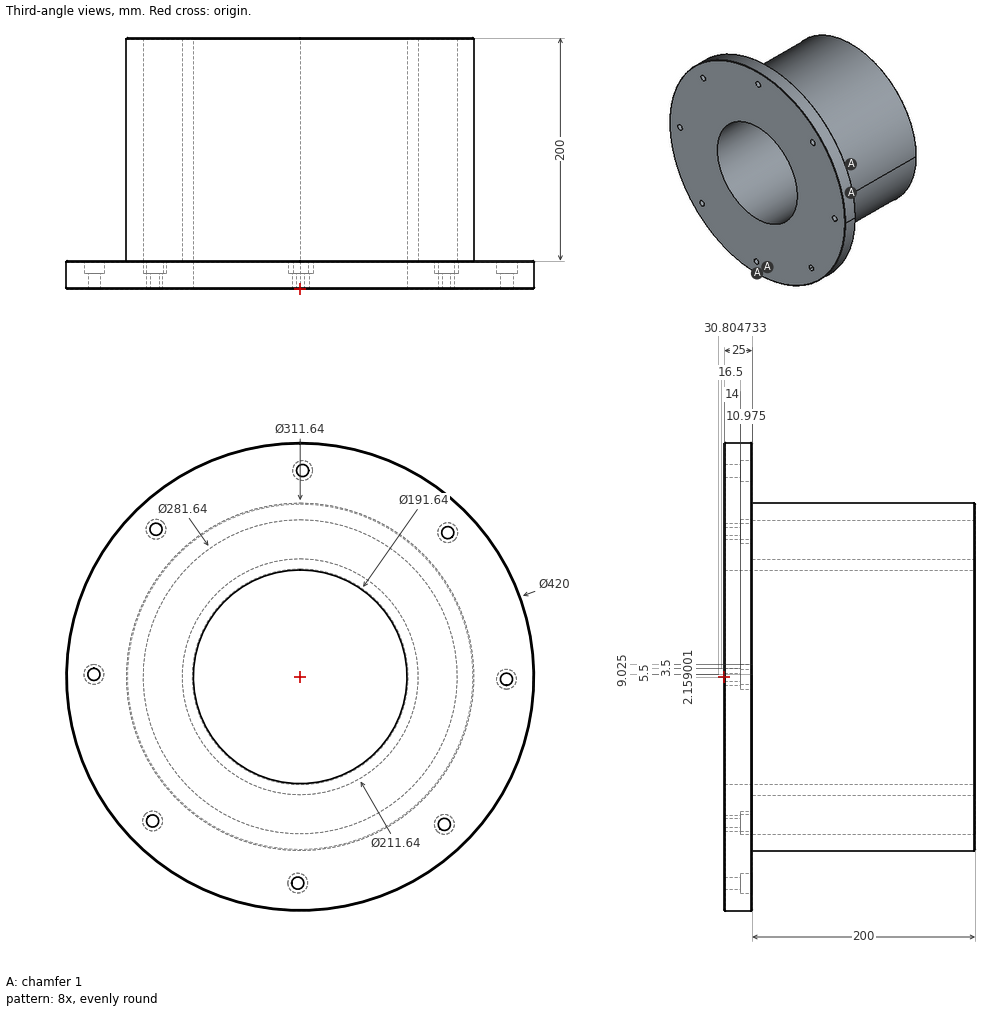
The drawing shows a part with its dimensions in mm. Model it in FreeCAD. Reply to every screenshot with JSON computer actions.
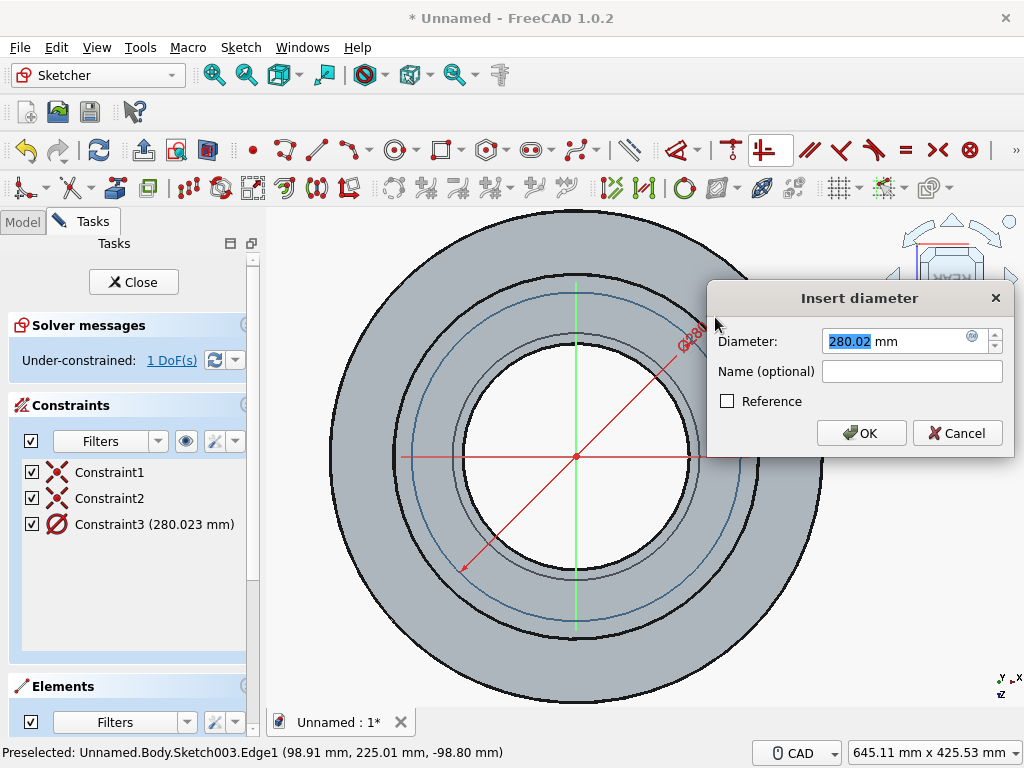
{"action": "type", "text": "281.64"}
{"action": "key", "text": "Return"}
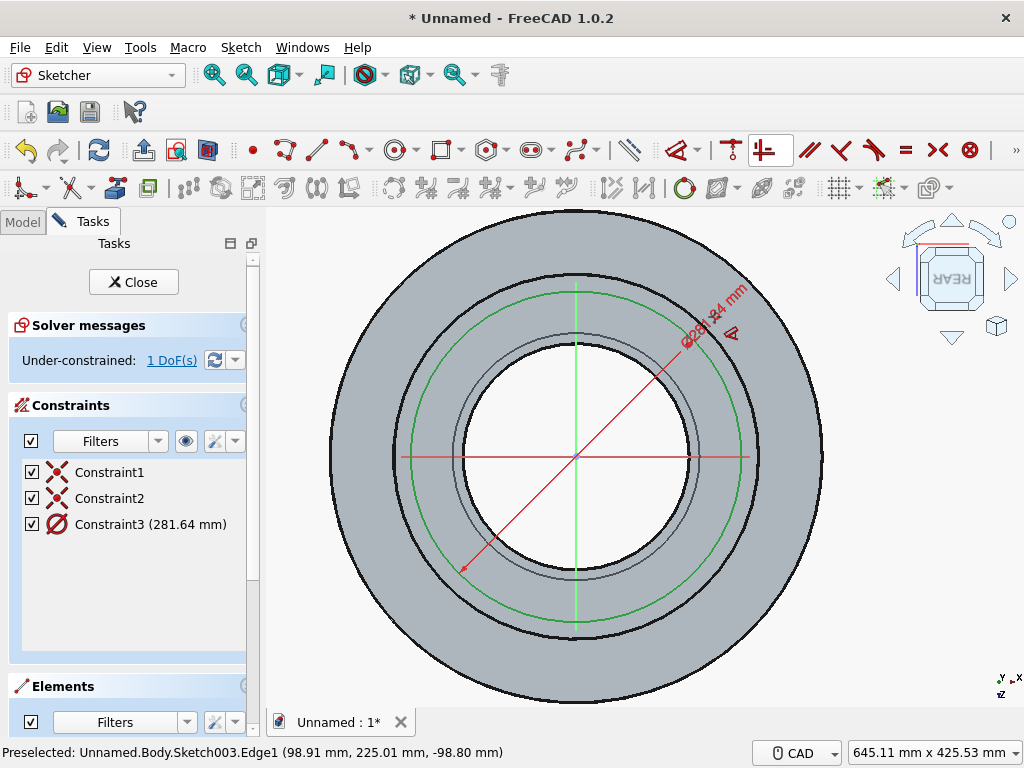
{"action": "left_click", "coordinate": [663, 369]}
{"action": "left_click", "coordinate": [747, 406]}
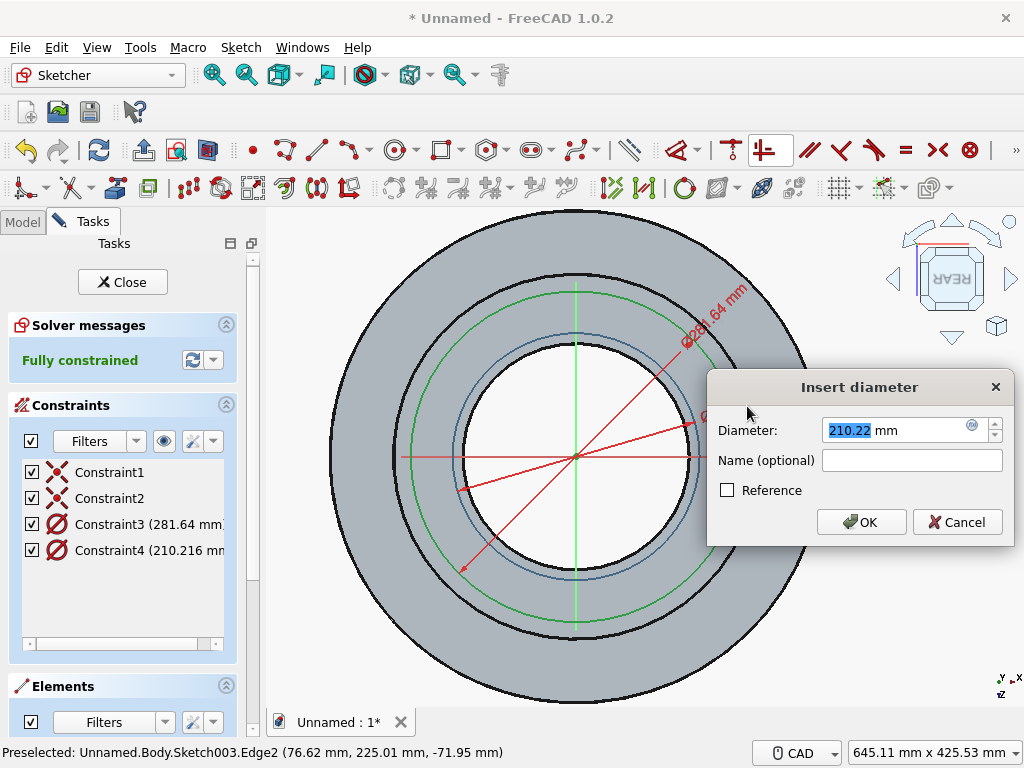
{"action": "type", "text": "211.64"}
{"action": "key", "text": "Return"}
{"action": "key", "text": "Escape"}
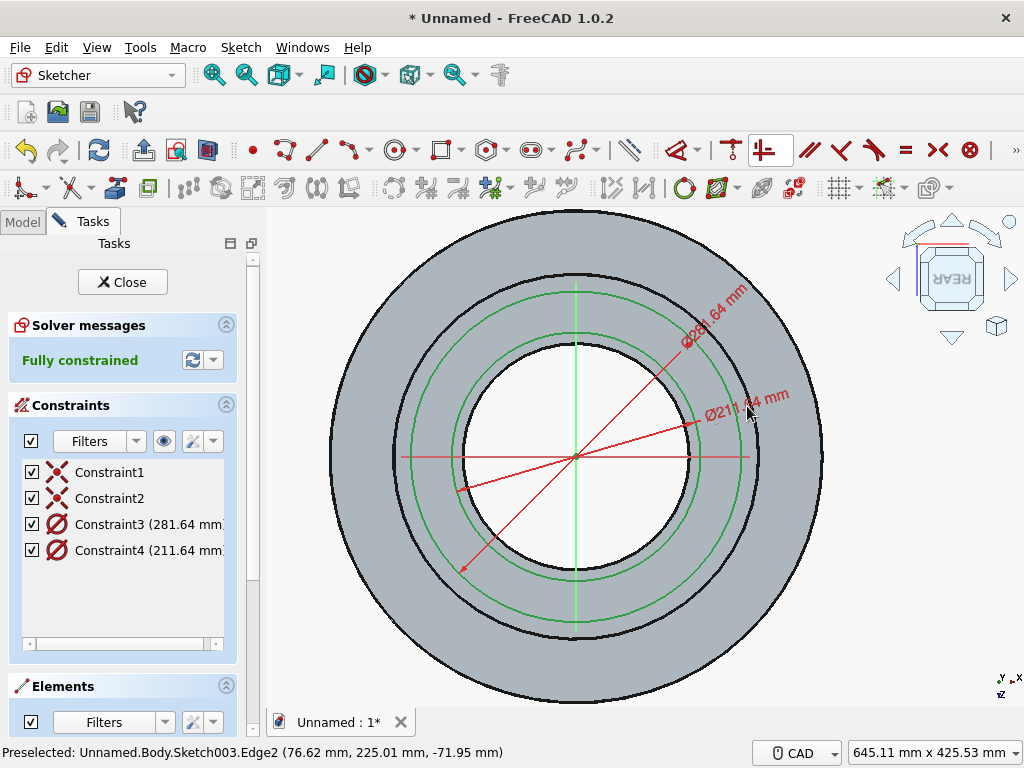
{"action": "left_click", "coordinate": [123, 282]}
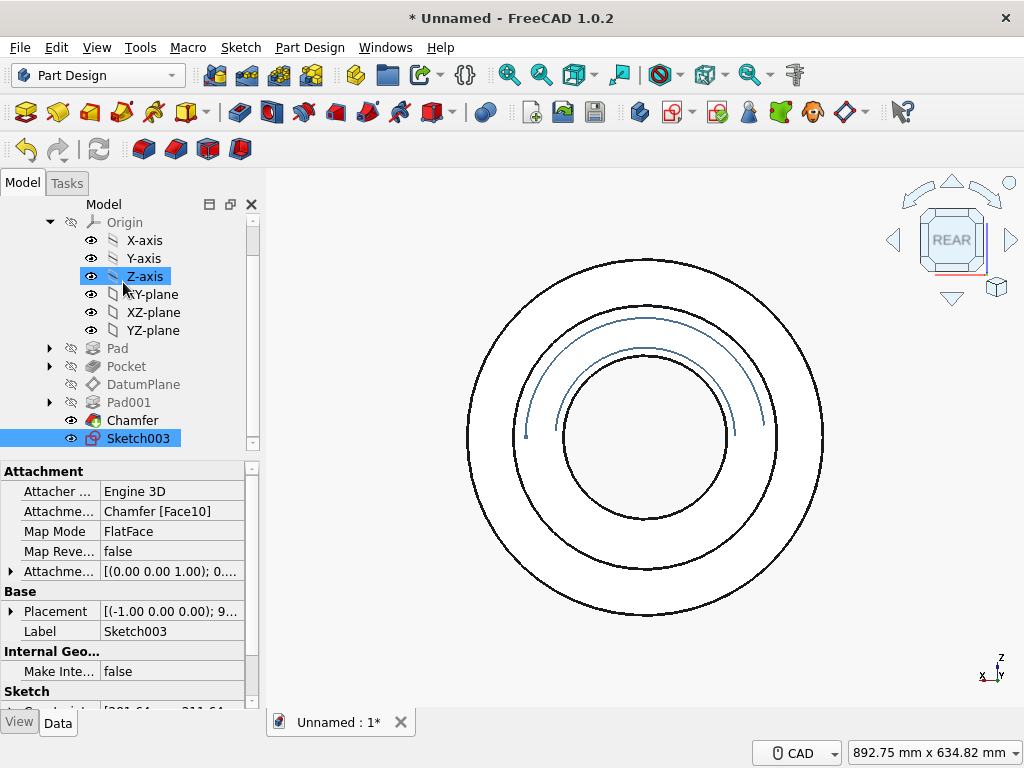
{"action": "left_click", "coordinate": [240, 112]}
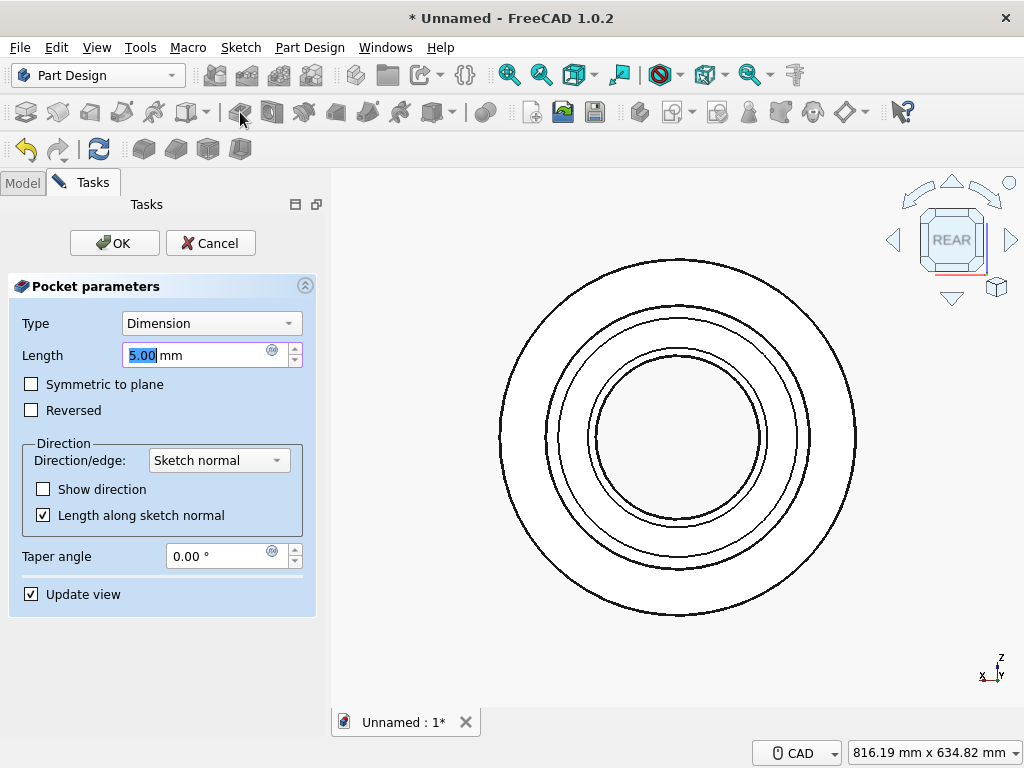
{"action": "type", "text": "200"}
{"action": "key", "text": "Tab"}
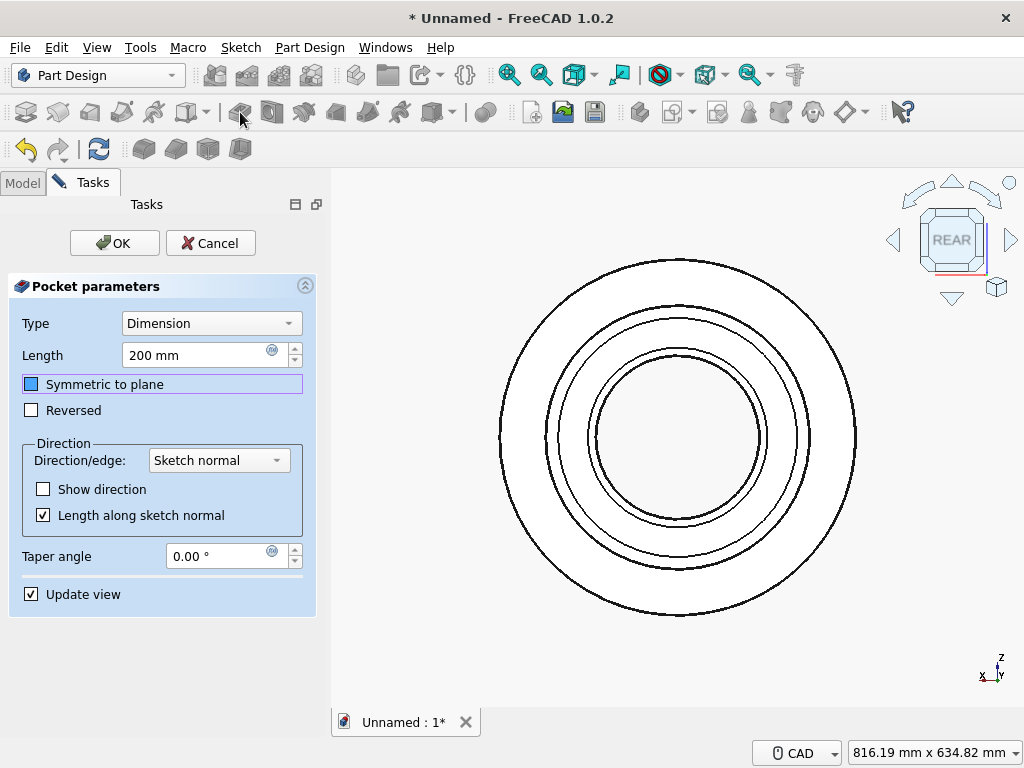
{"action": "left_click", "coordinate": [115, 243]}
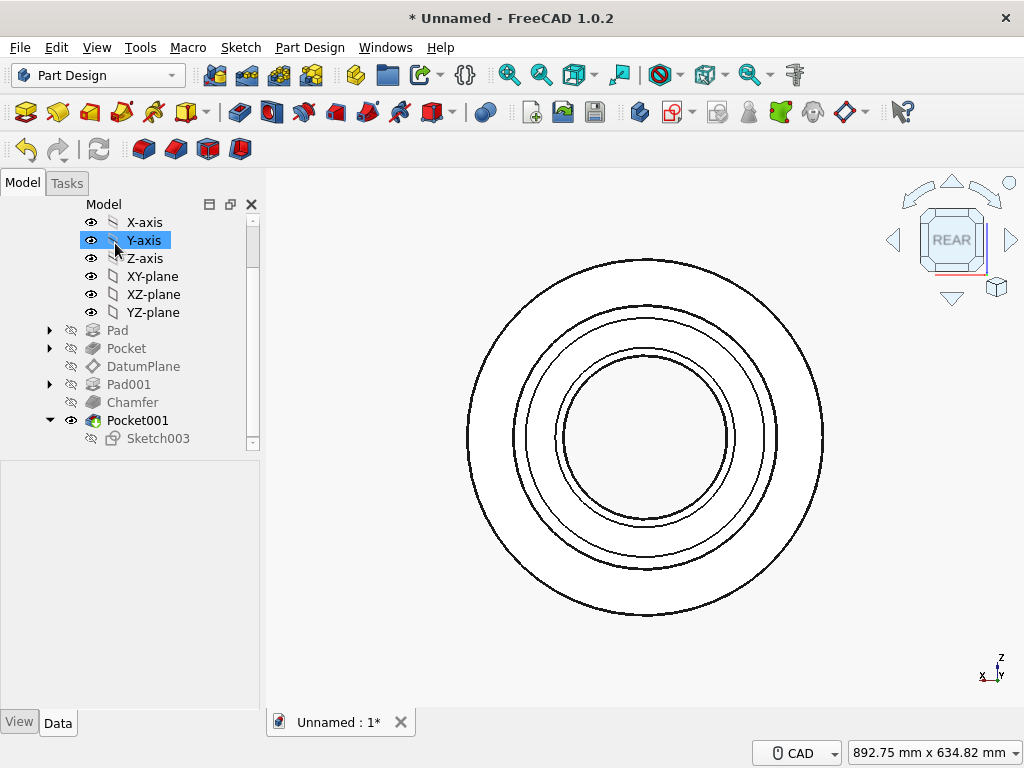
{"action": "scroll", "coordinate": [160, 326], "scroll_direction": "down", "scroll_amount": 3}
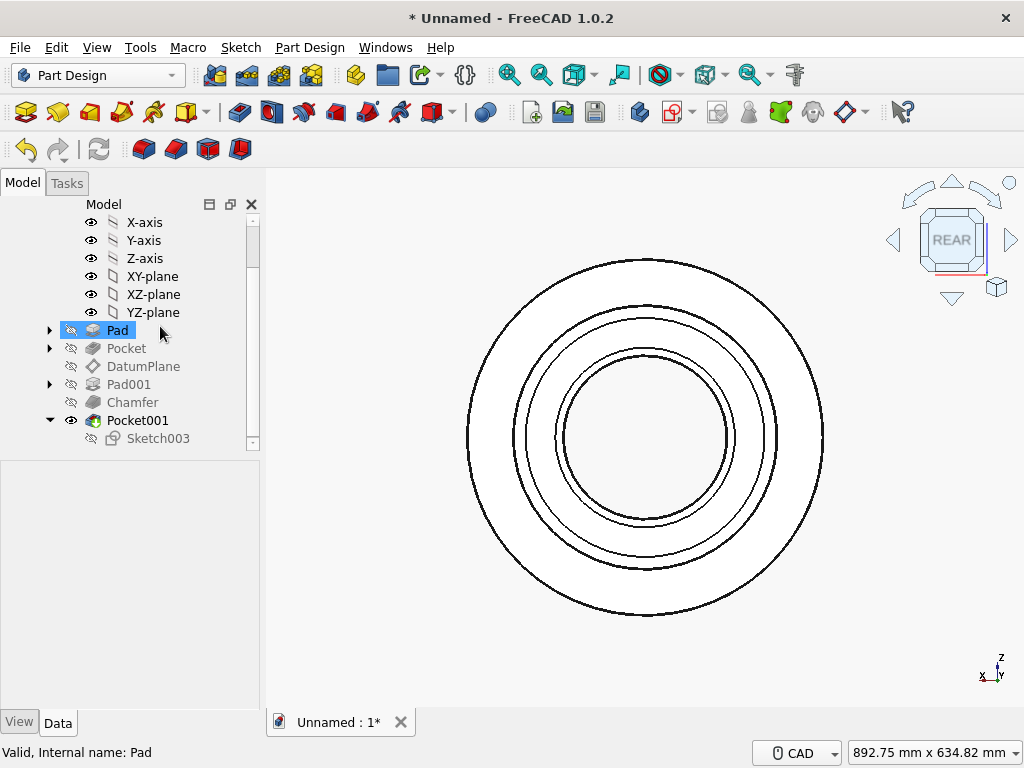
{"action": "scroll", "coordinate": [160, 326], "scroll_direction": "up", "scroll_amount": 15}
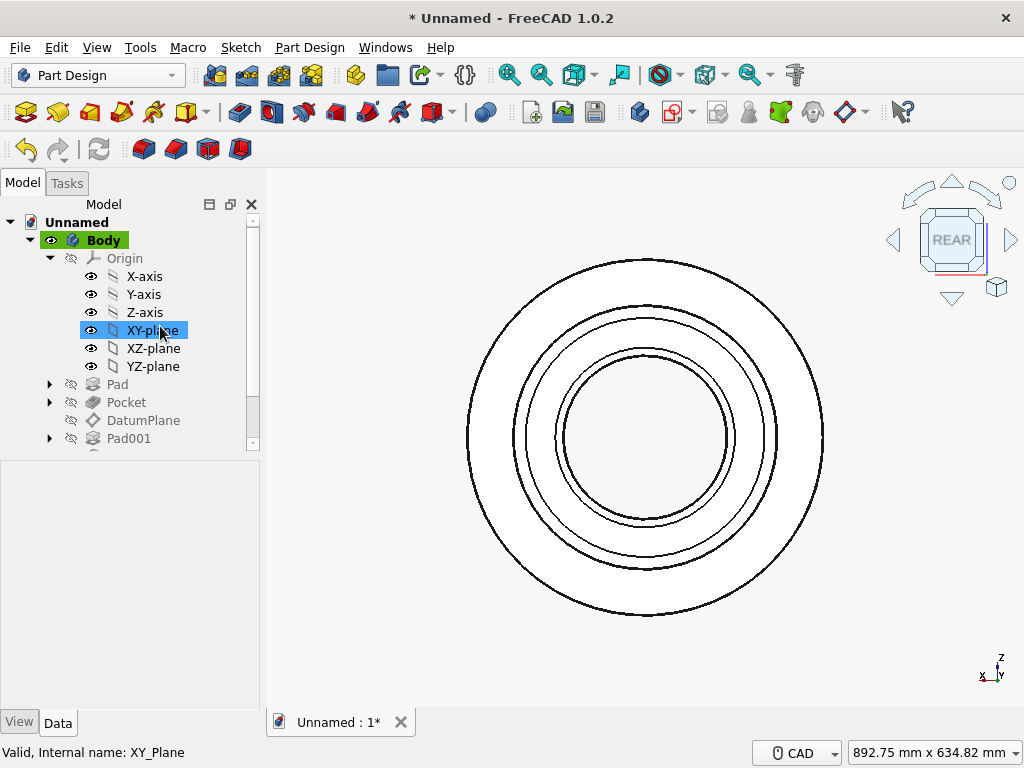
{"action": "left_click", "coordinate": [136, 366]}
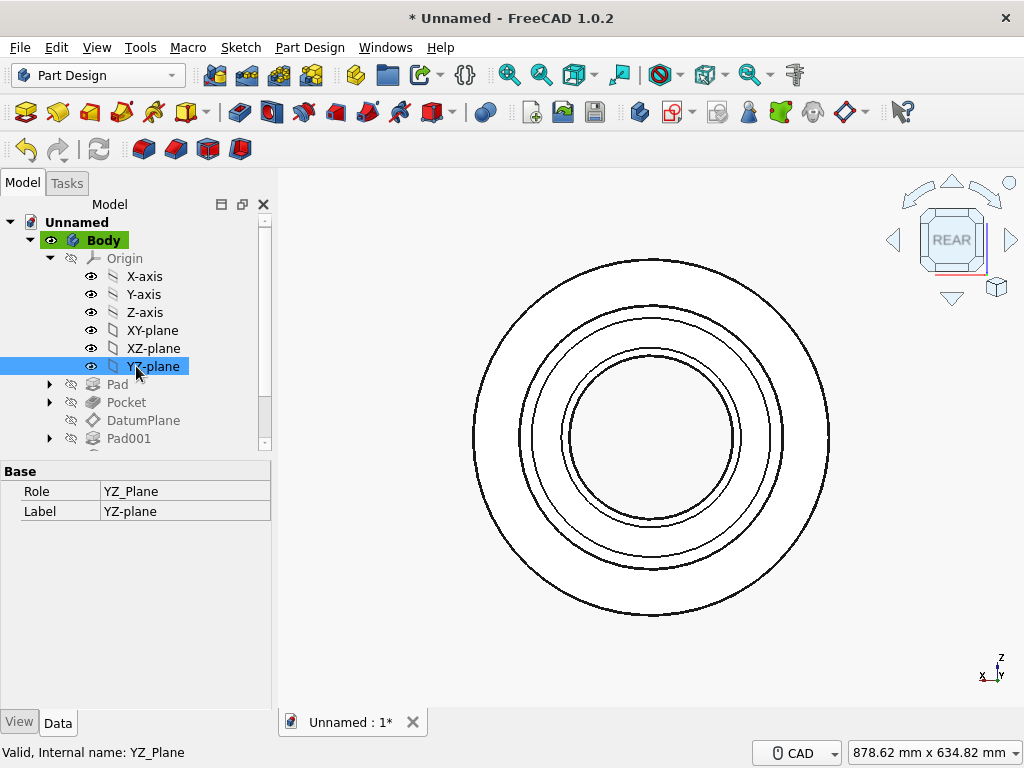
{"action": "left_click", "coordinate": [846, 112]}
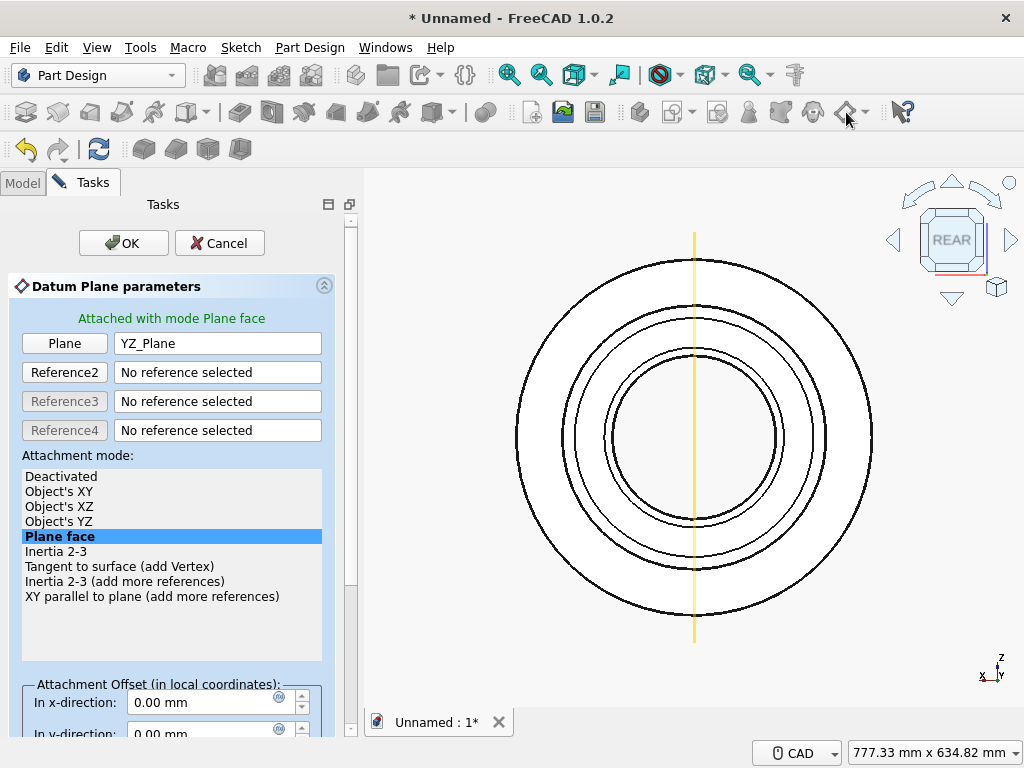
{"action": "scroll", "coordinate": [351, 475], "scroll_direction": "down", "scroll_amount": 2}